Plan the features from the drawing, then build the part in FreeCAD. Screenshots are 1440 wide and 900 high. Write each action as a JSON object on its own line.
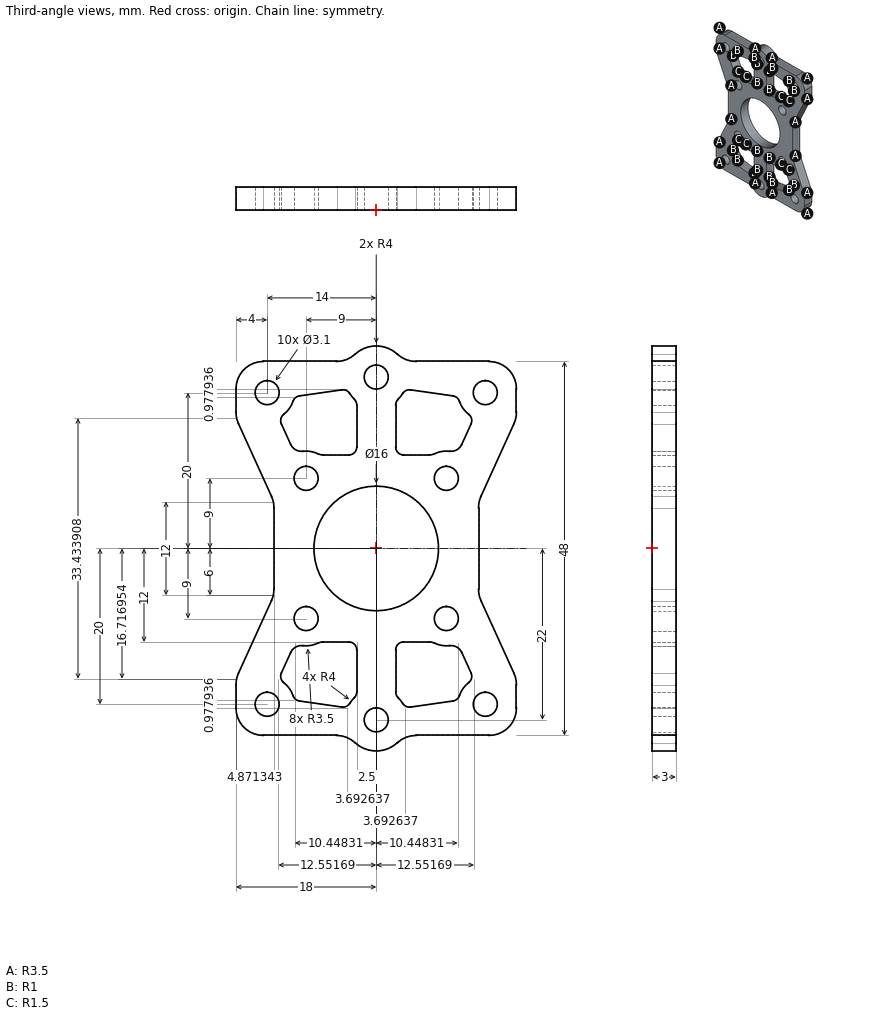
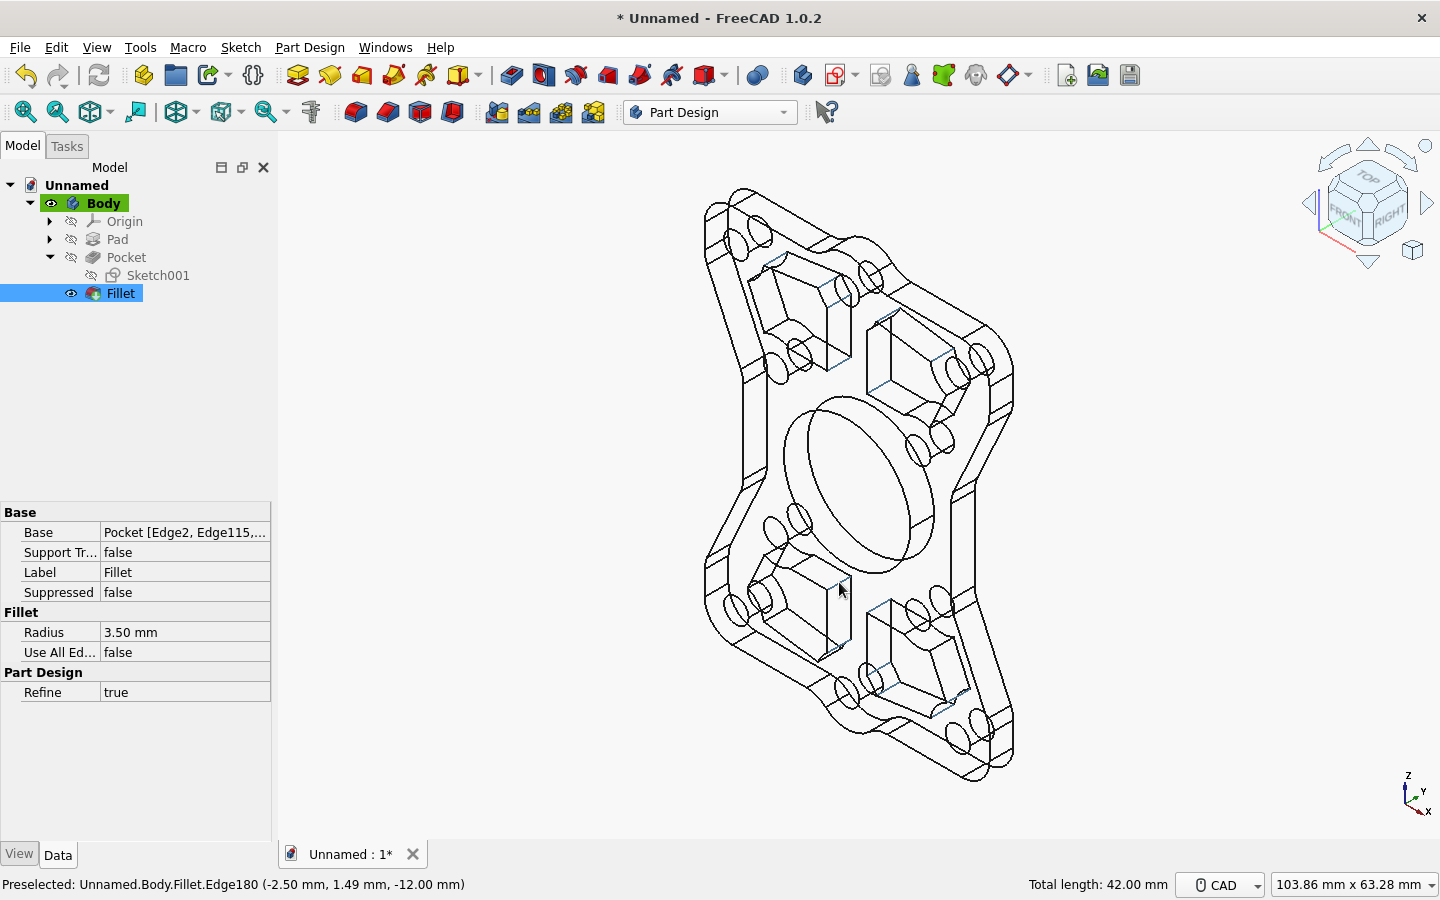
{"action": "left_click", "coordinate": [760, 580], "text": "ctrl"}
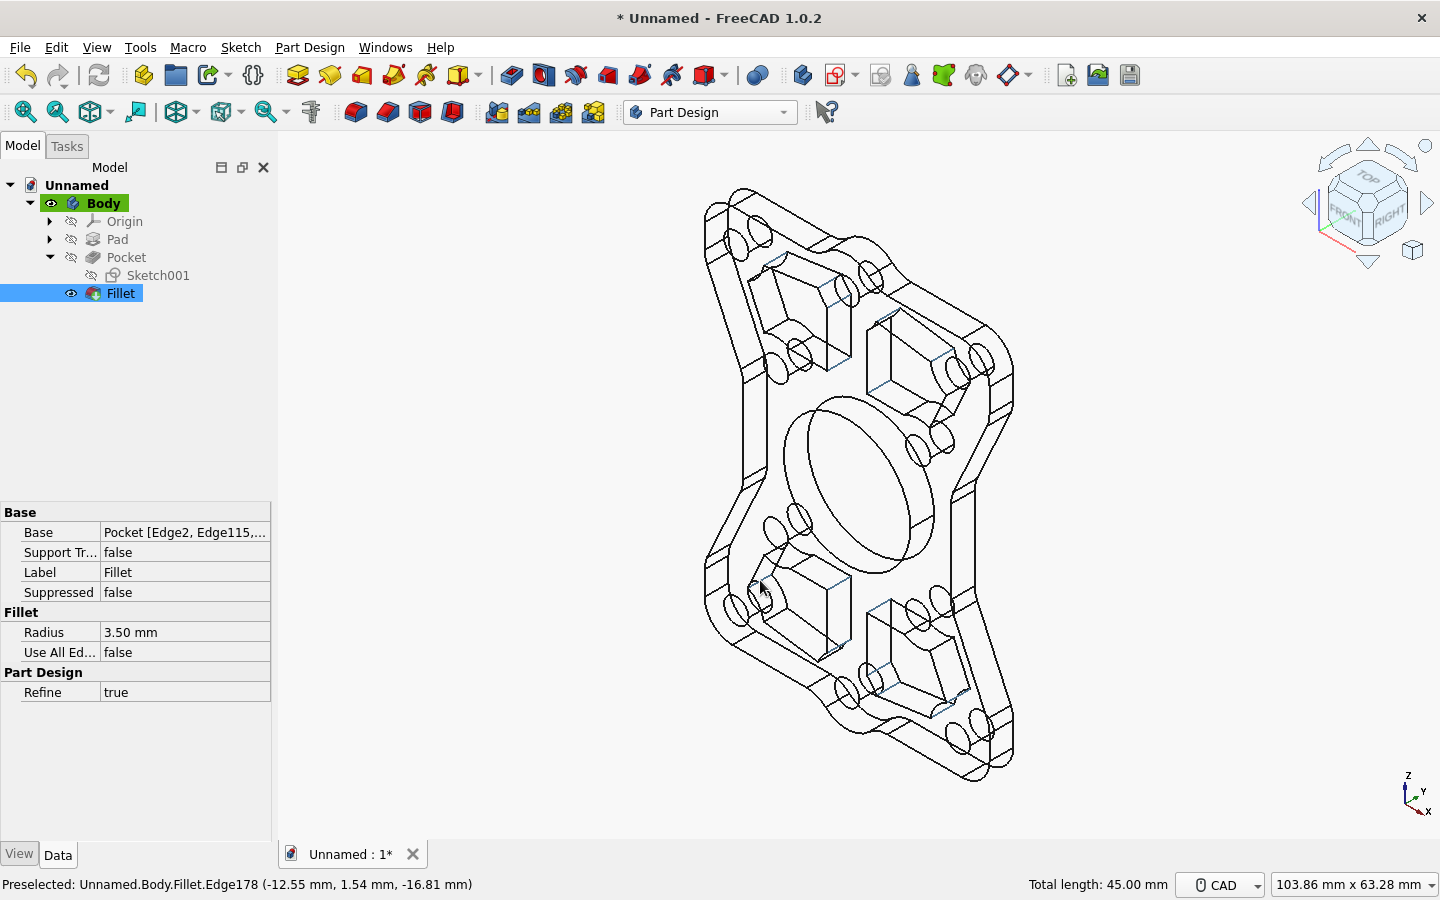
{"action": "left_click", "coordinate": [776, 614], "text": "ctrl"}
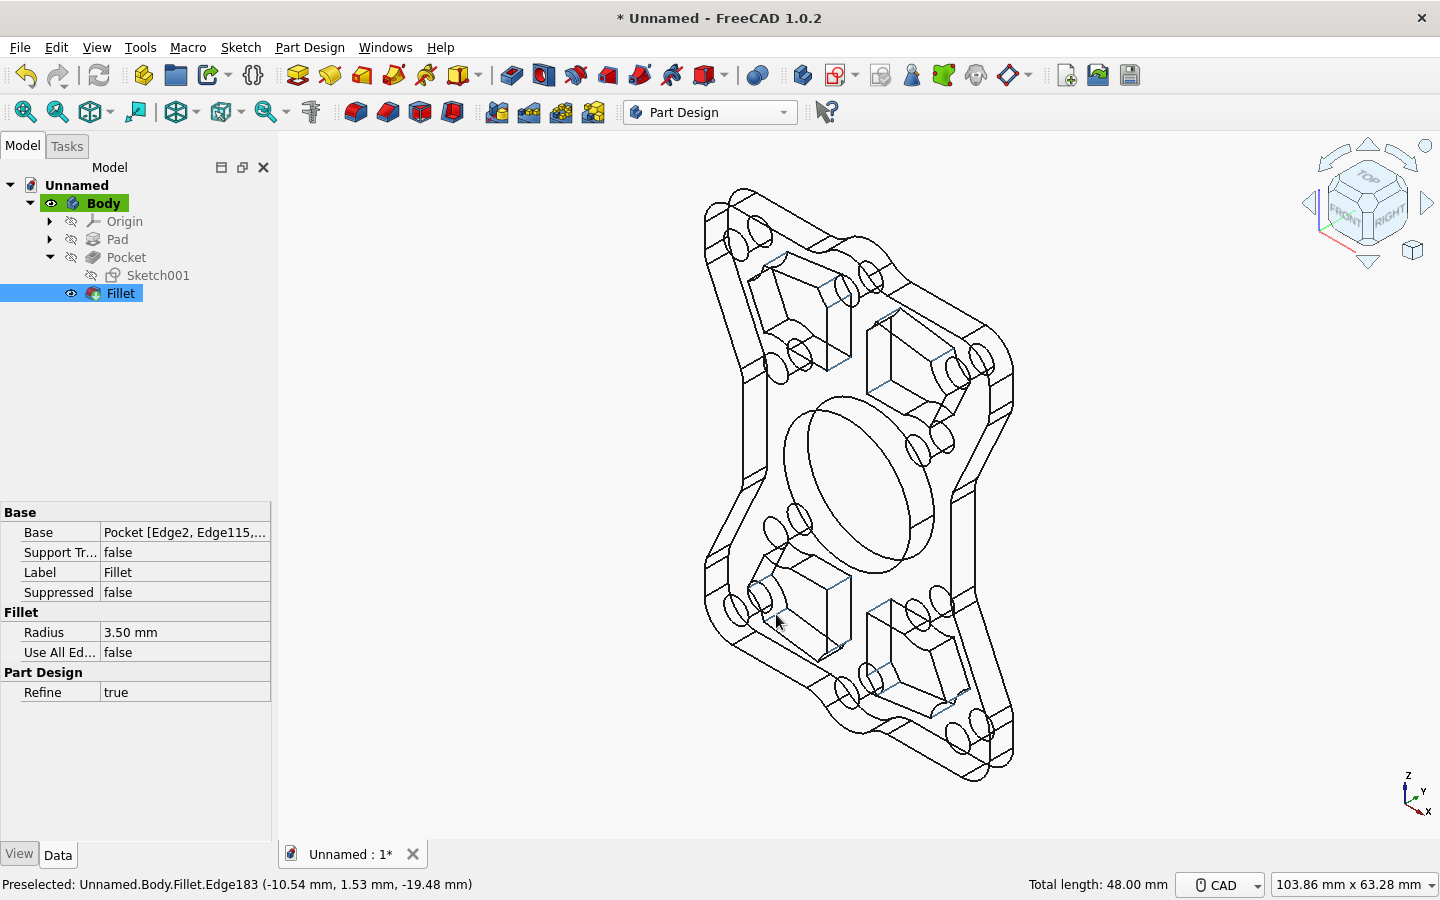
{"action": "key", "text": "2"}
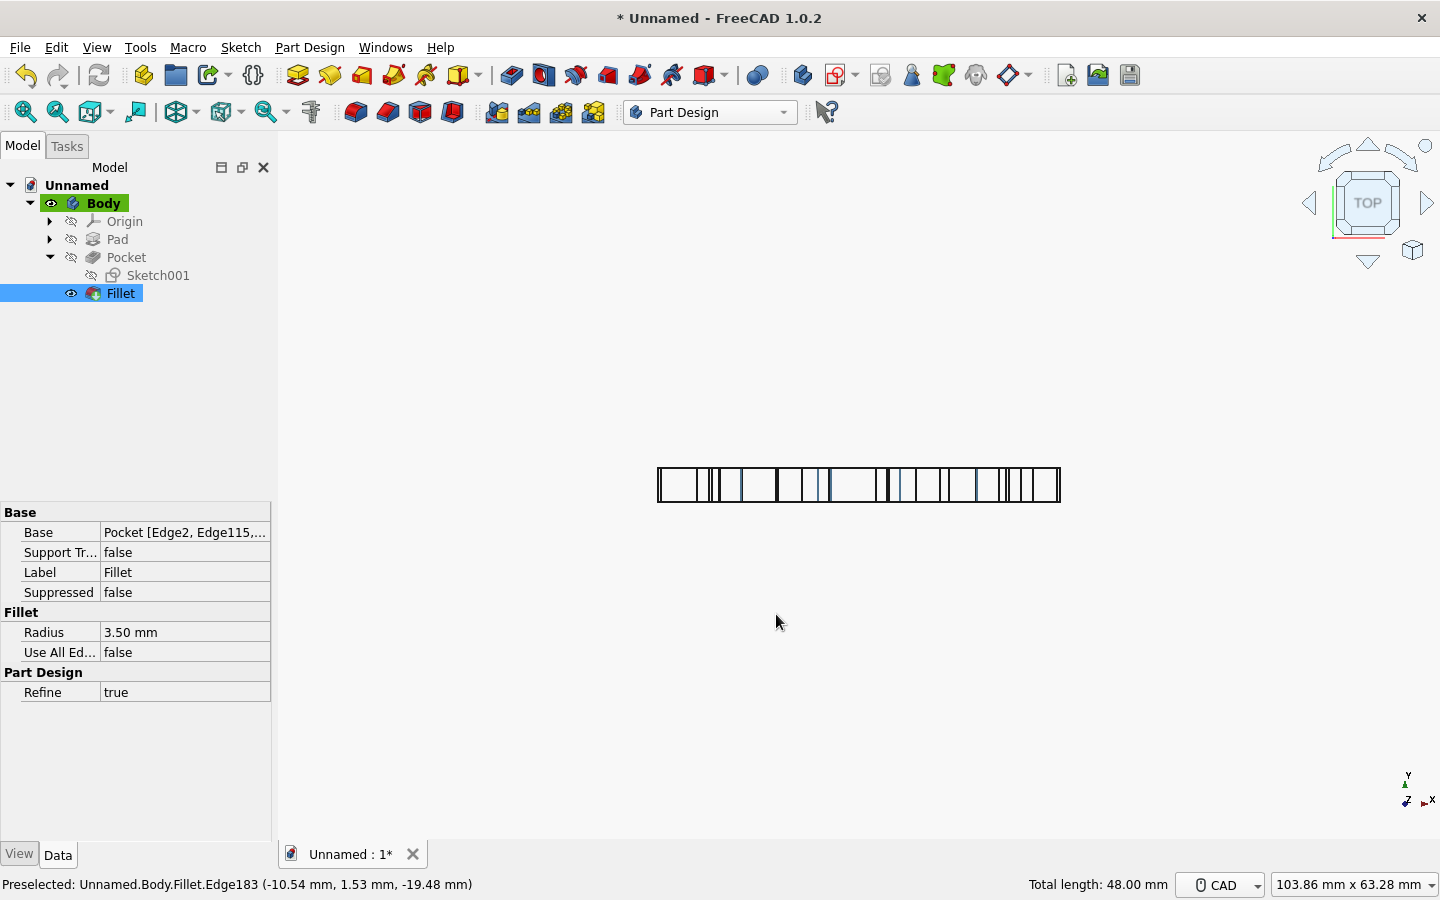
{"action": "left_click", "coordinate": [26, 112]}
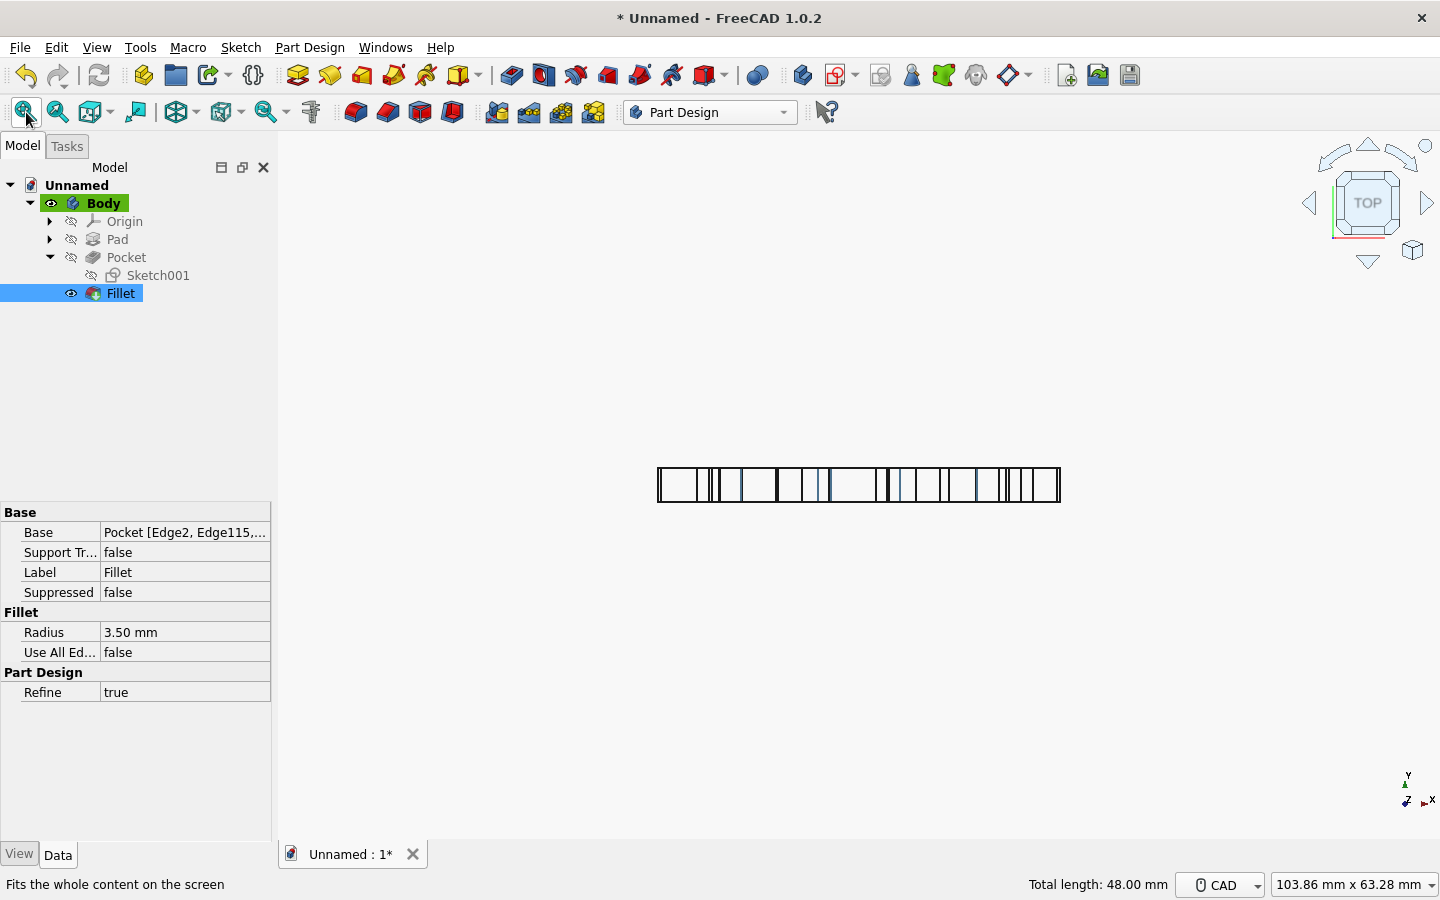
{"action": "left_click", "coordinate": [999, 484], "text": "ctrl"}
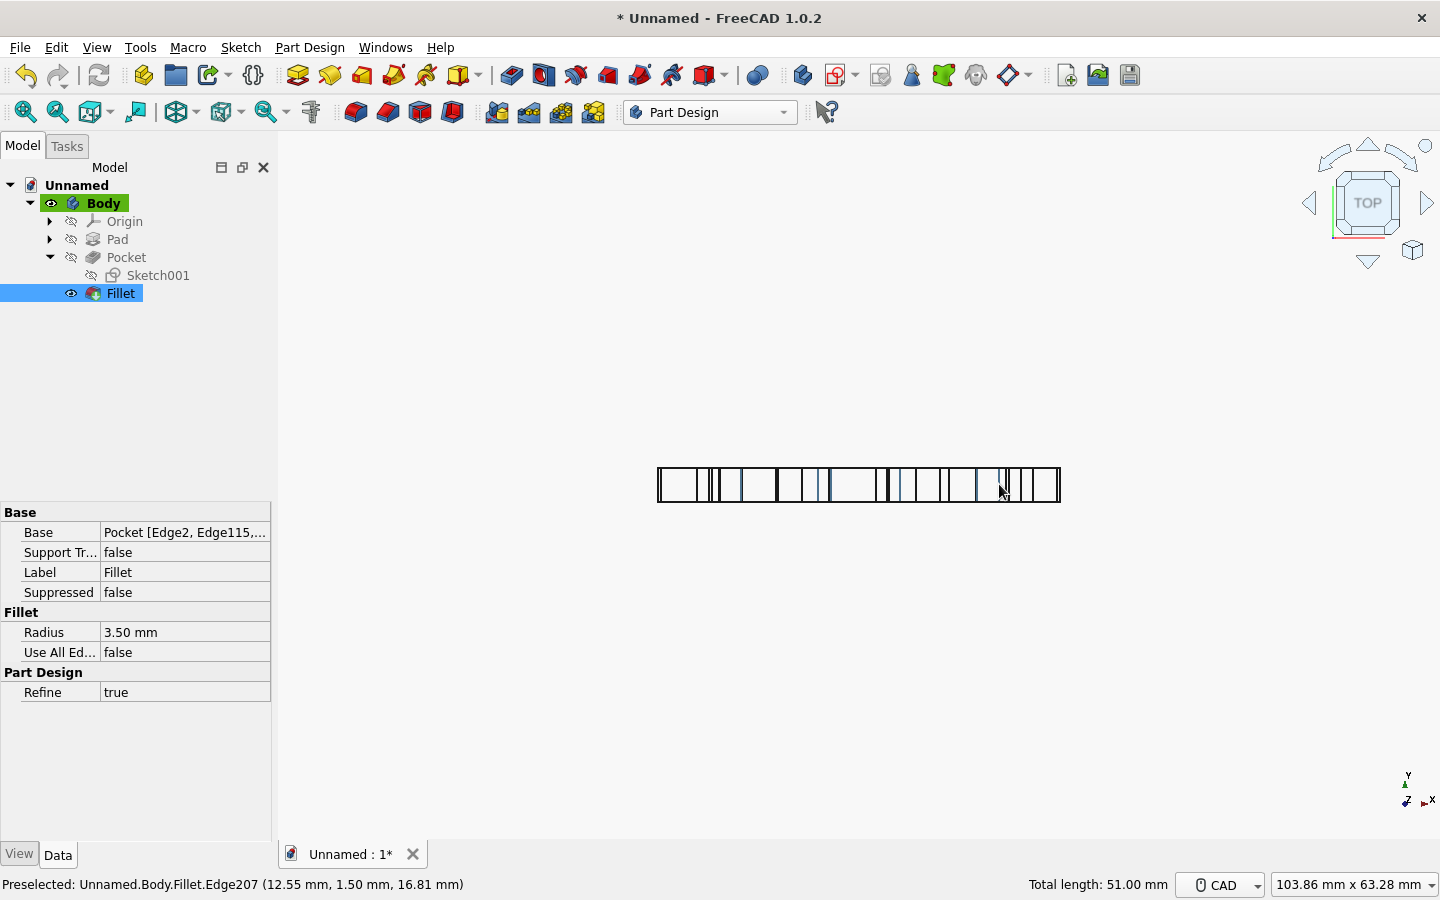
{"action": "key", "text": "1"}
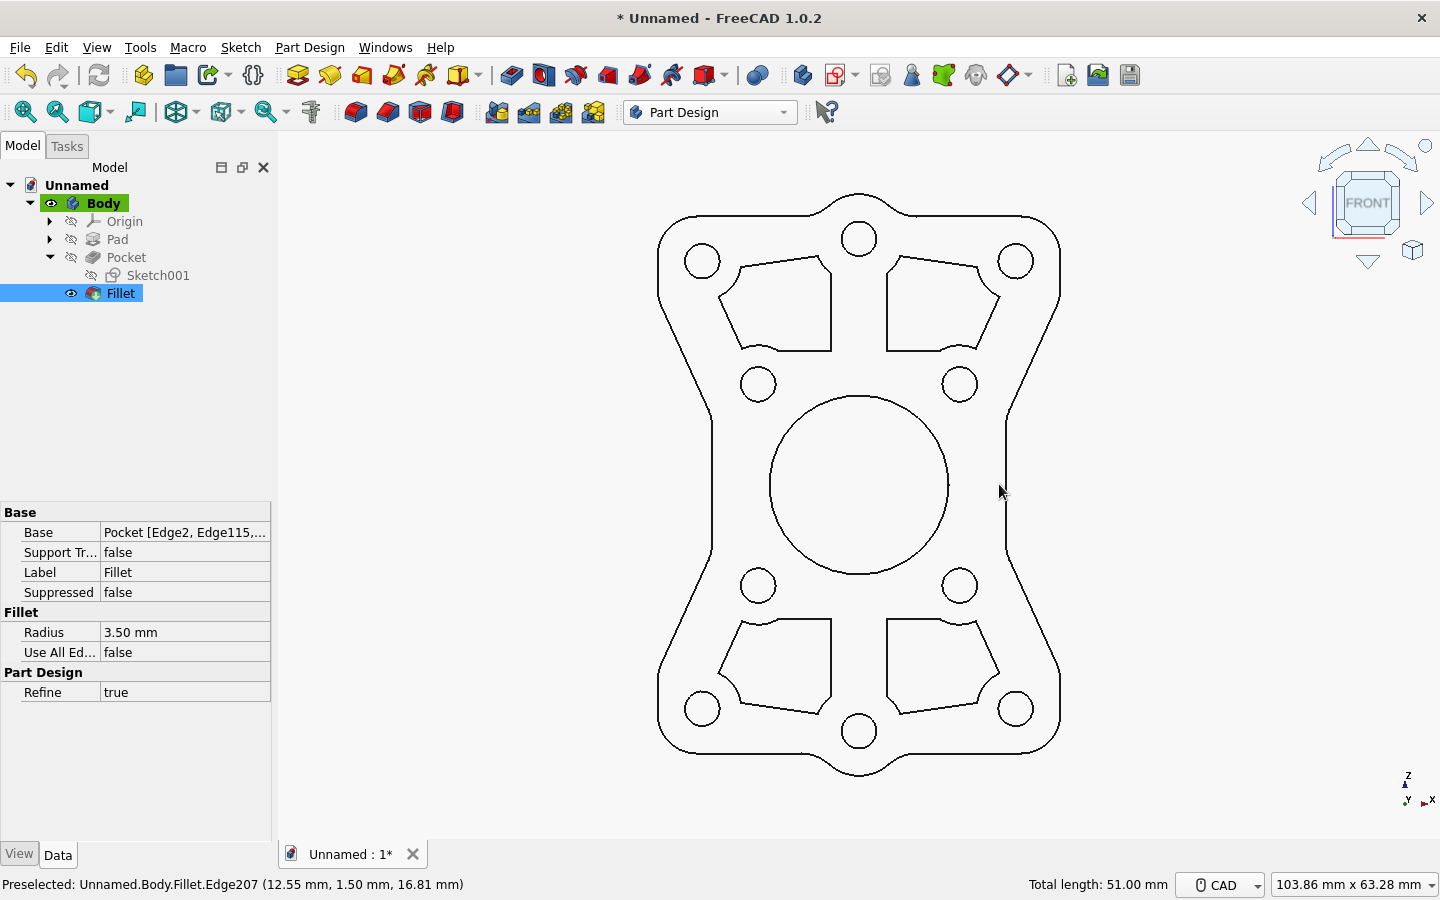
{"action": "key", "text": "3"}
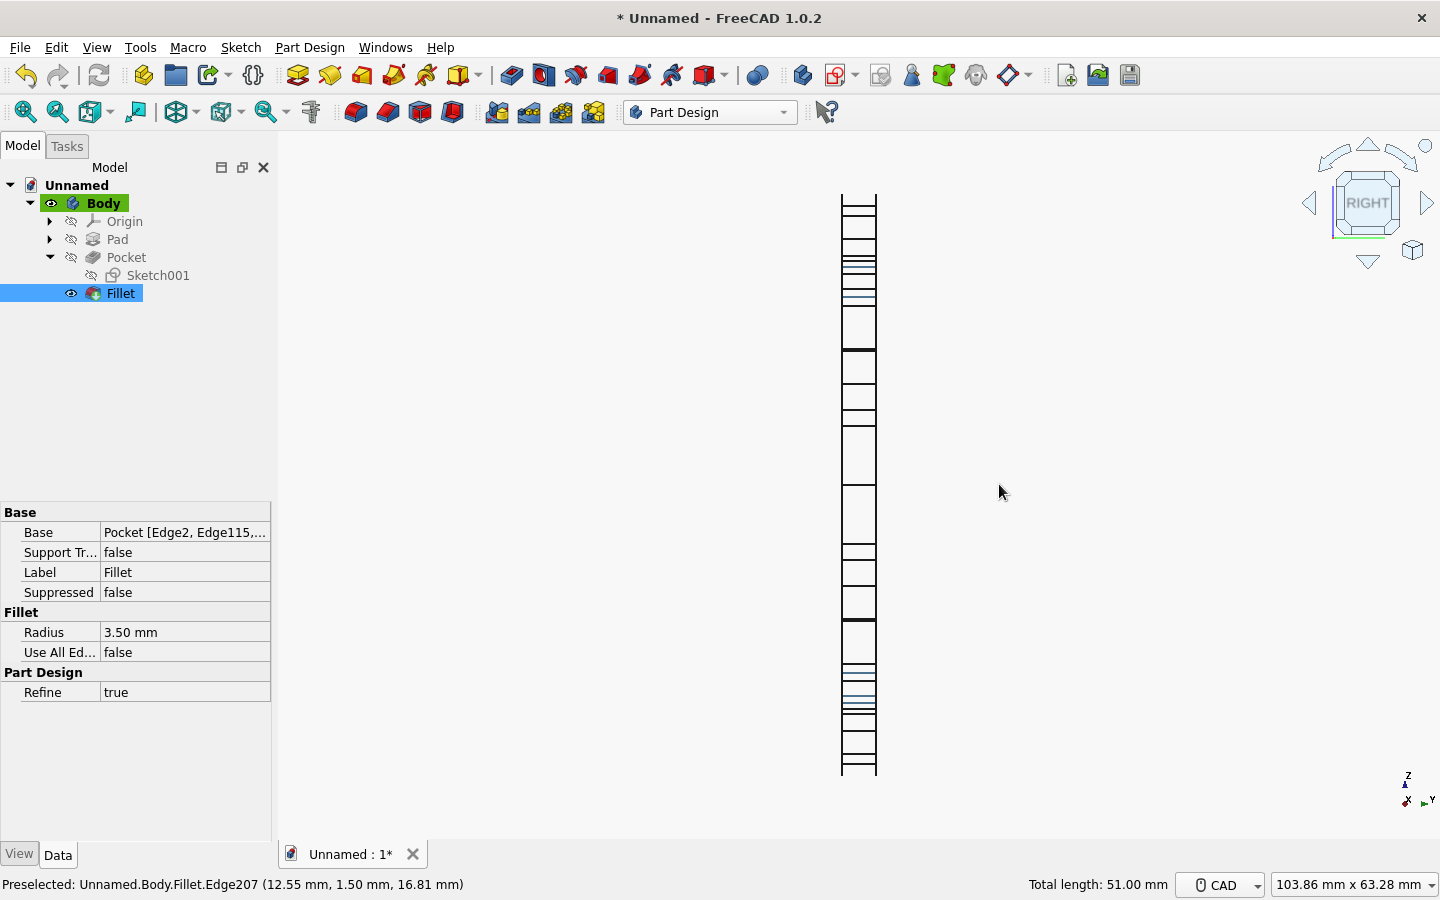
{"action": "left_click", "coordinate": [859, 273], "text": "ctrl"}